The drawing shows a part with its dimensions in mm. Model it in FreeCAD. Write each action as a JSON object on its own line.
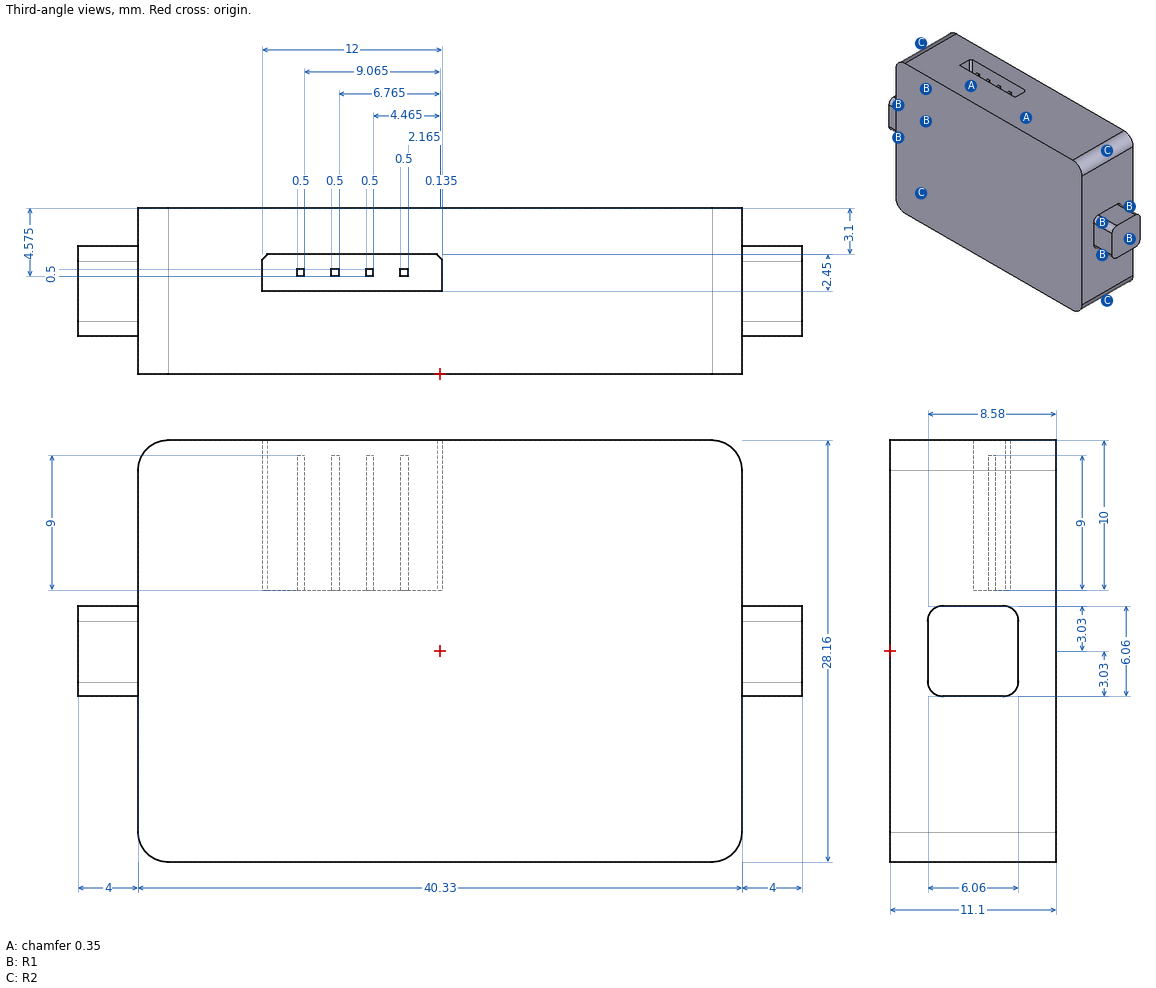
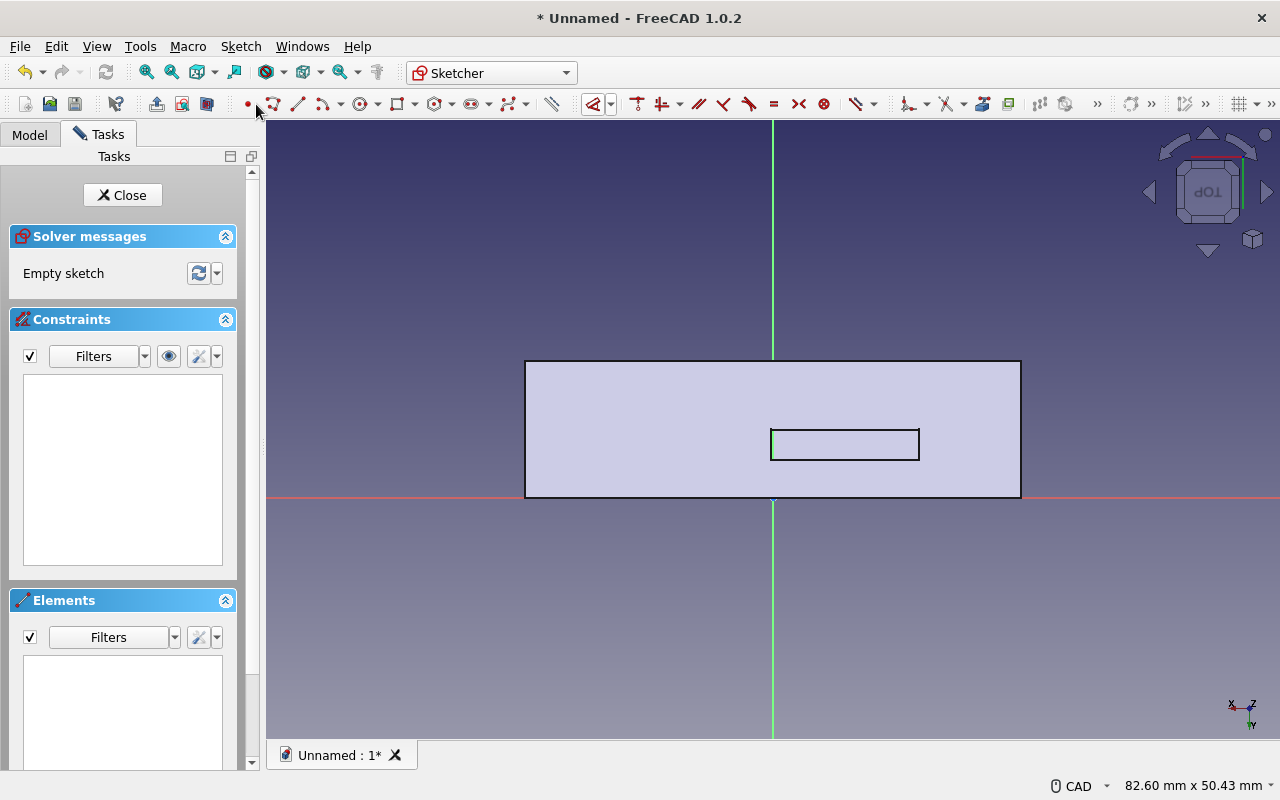
{"action": "scroll", "coordinate": [838, 445], "scroll_direction": "up", "scroll_amount": 15}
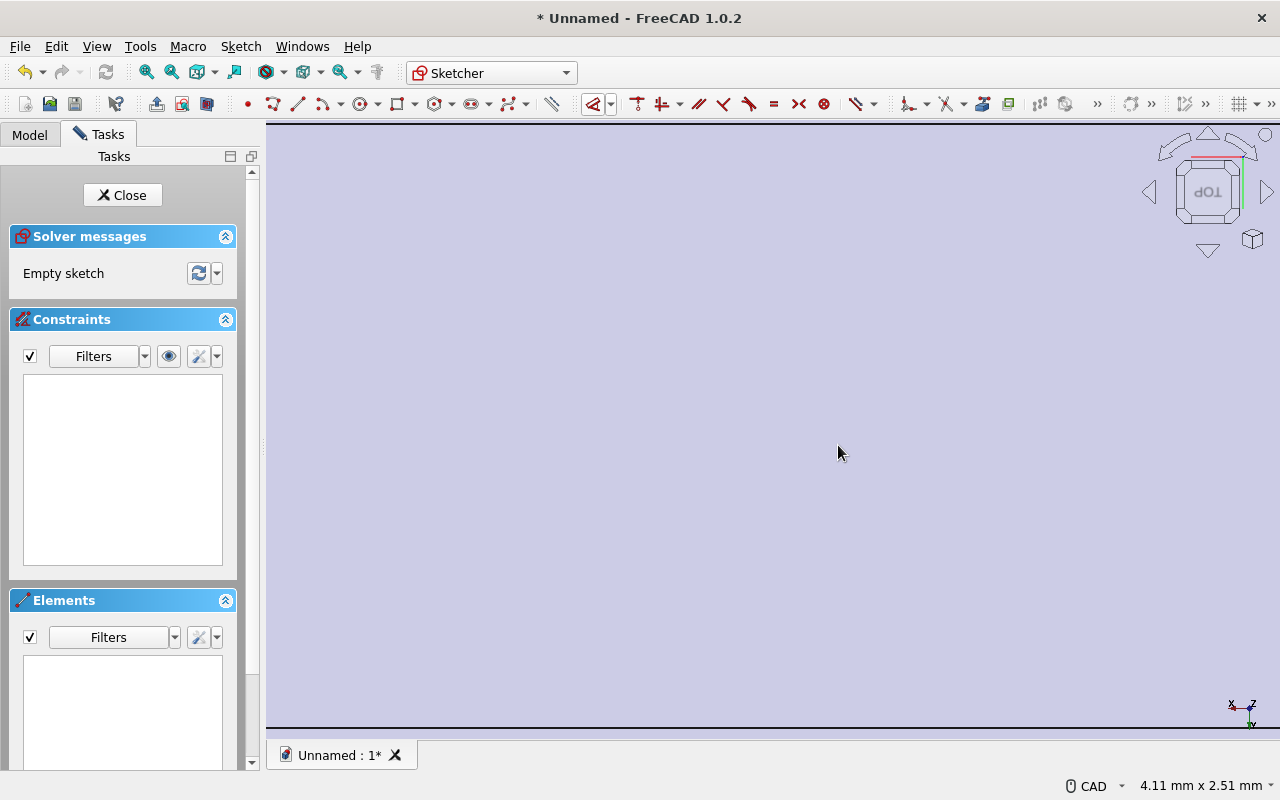
{"action": "scroll", "coordinate": [675, 424], "scroll_direction": "up", "scroll_amount": 6}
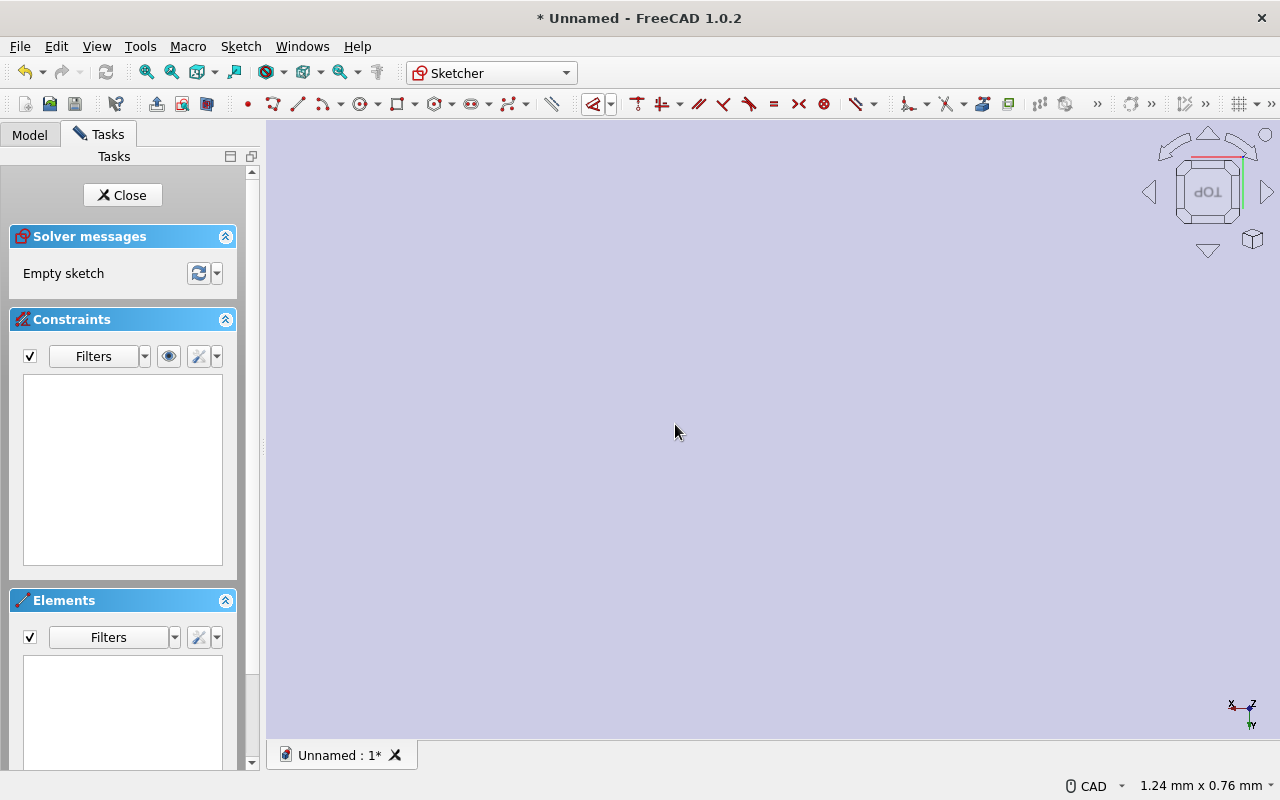
{"action": "key", "text": "g r"}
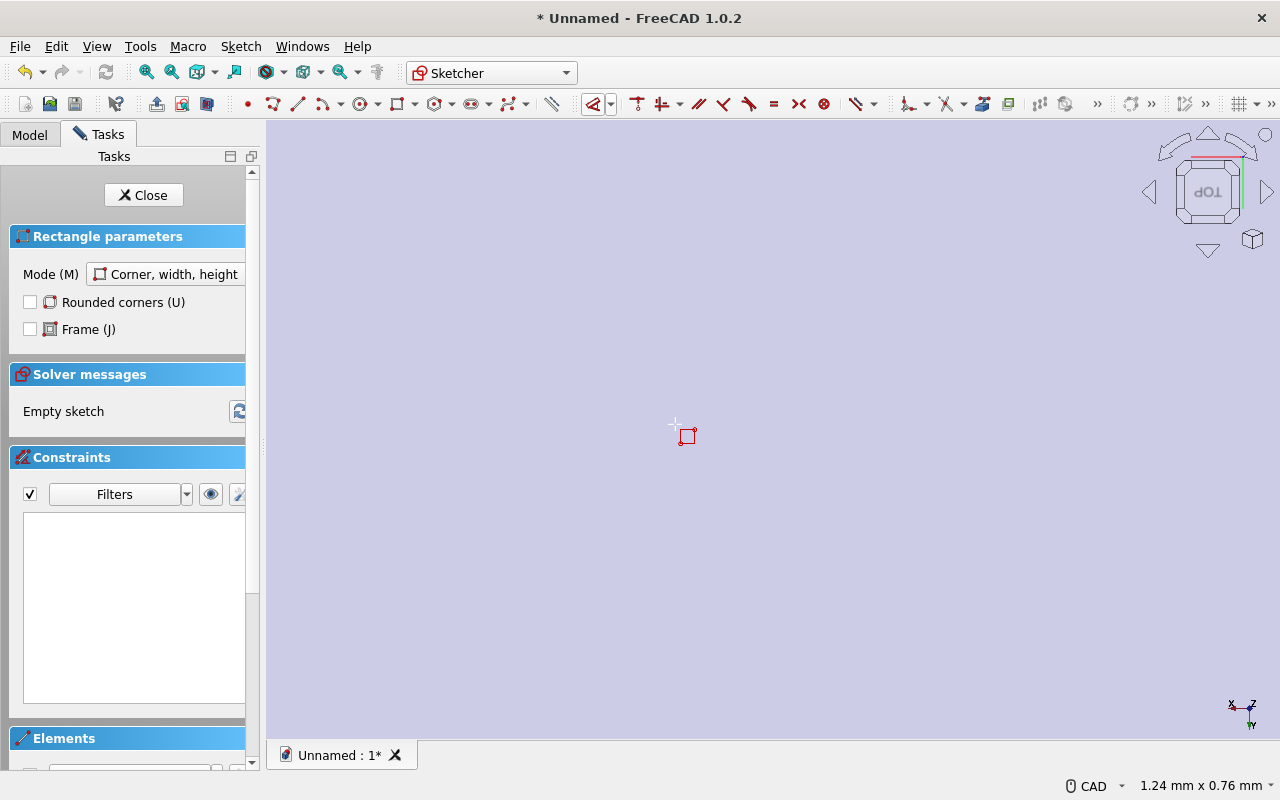
{"action": "left_click", "coordinate": [500, 224]}
{"action": "mouse_move", "coordinate": [909, 633]}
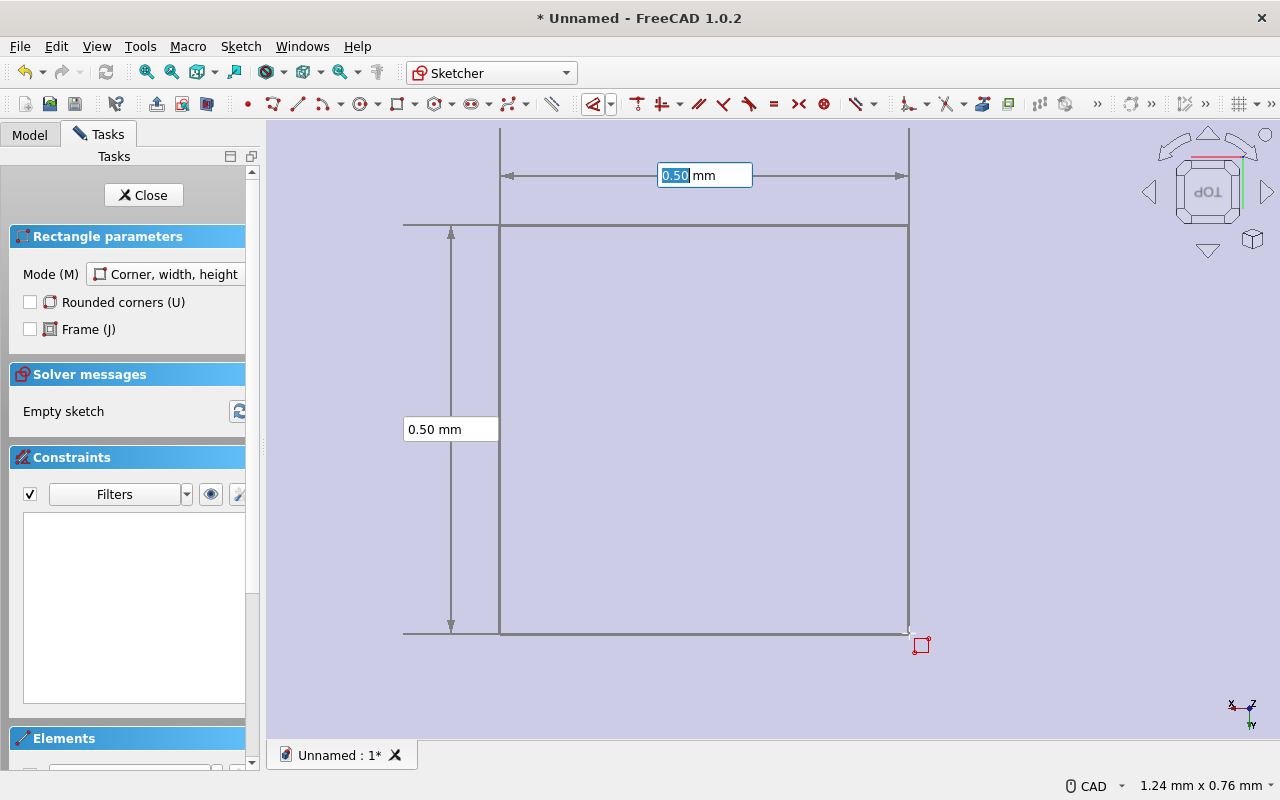
{"action": "type", "text": "0.5"}
{"action": "key", "text": "Tab"}
{"action": "type", "text": "0.5"}
{"action": "key", "text": "Return"}
{"action": "key", "text": "Escape"}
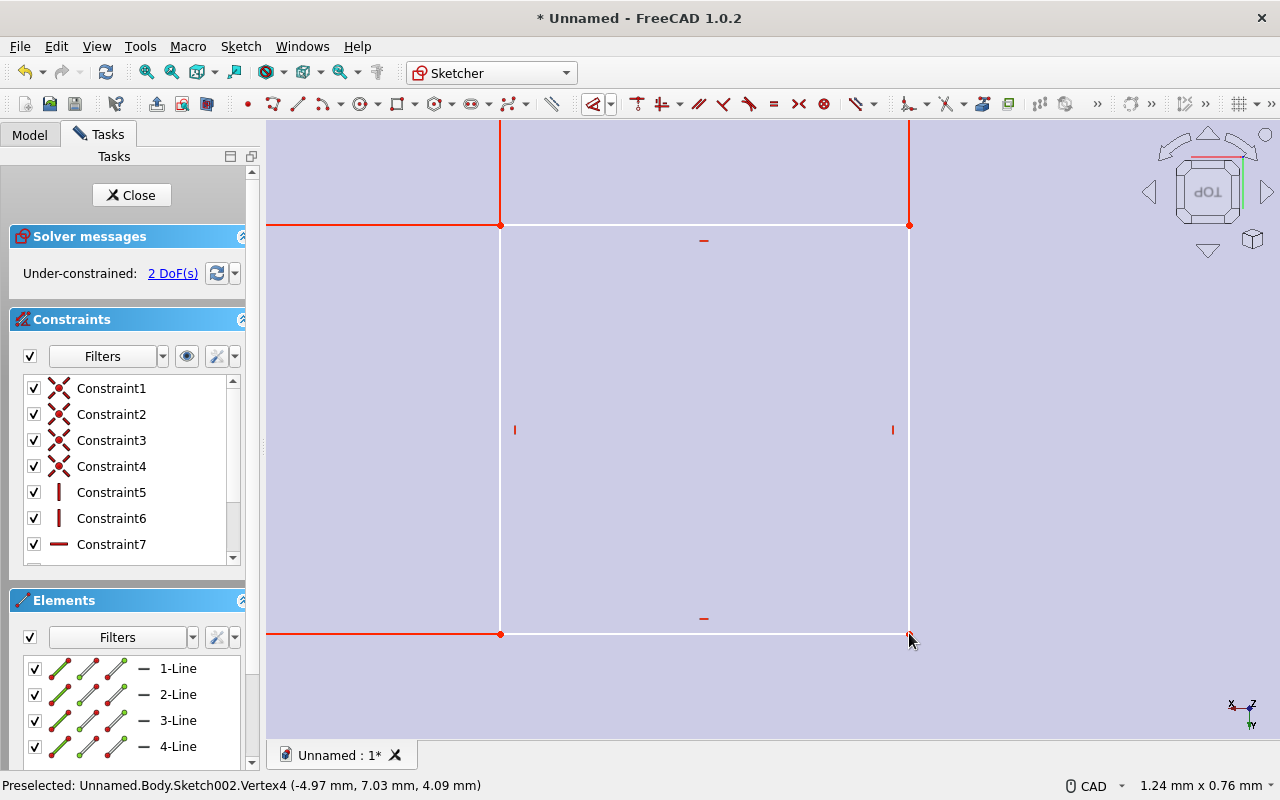
{"action": "left_click", "coordinate": [592, 104]}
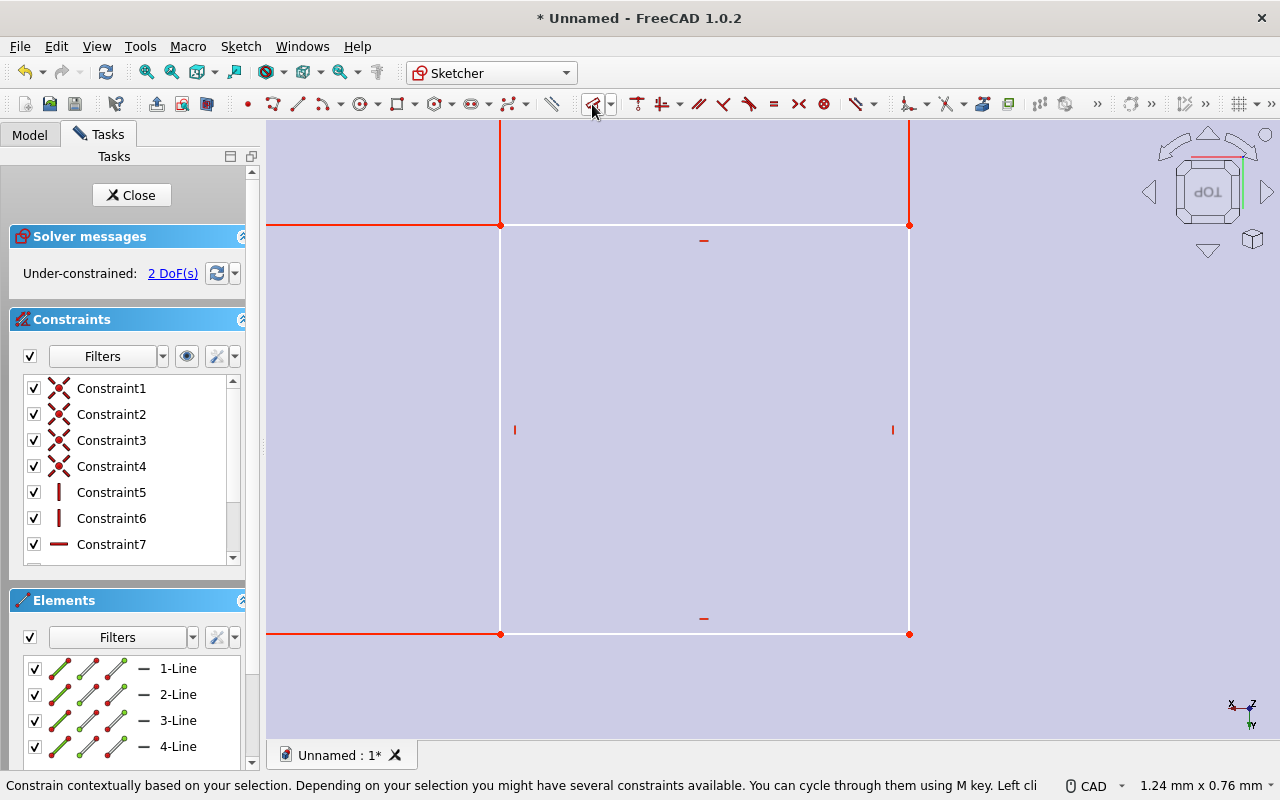
{"action": "left_click", "coordinate": [500, 225]}
{"action": "left_click", "coordinate": [397, 191]}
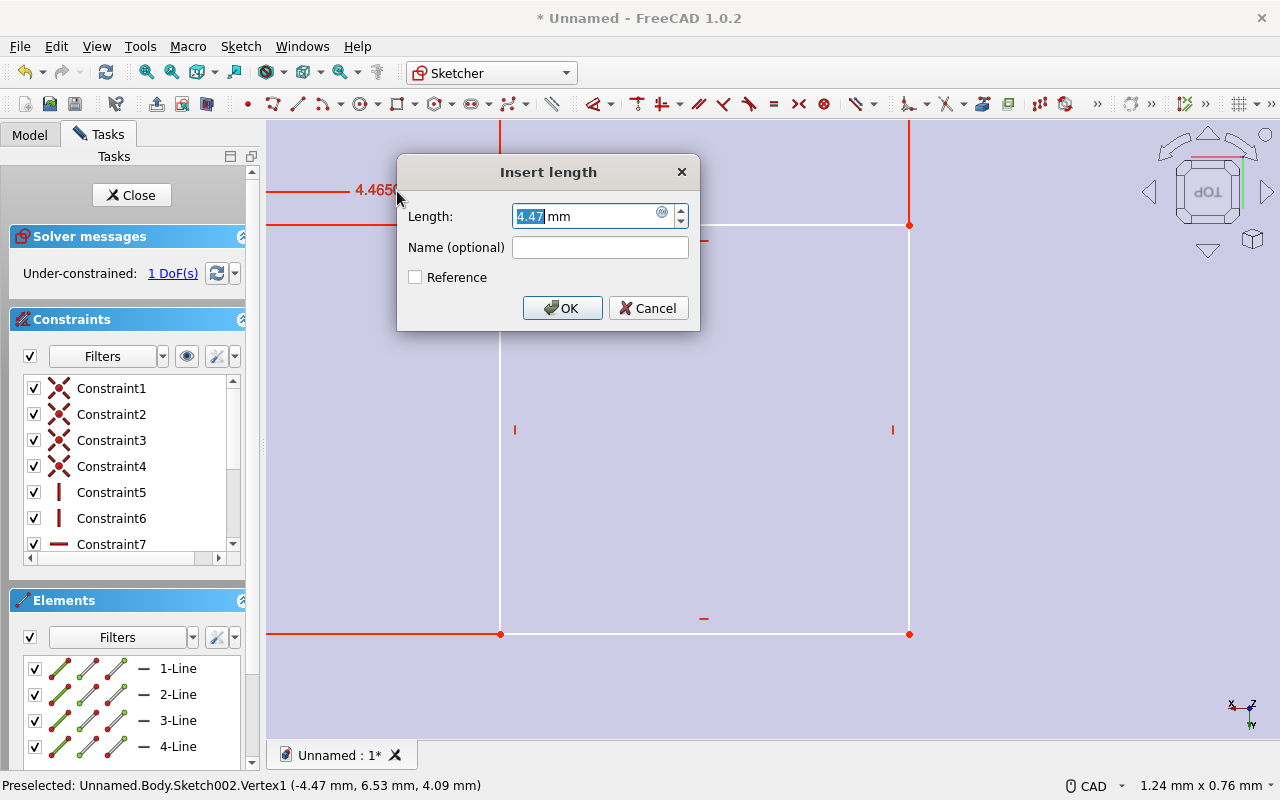
{"action": "type", "text": "4.465"}
{"action": "key", "text": "Return"}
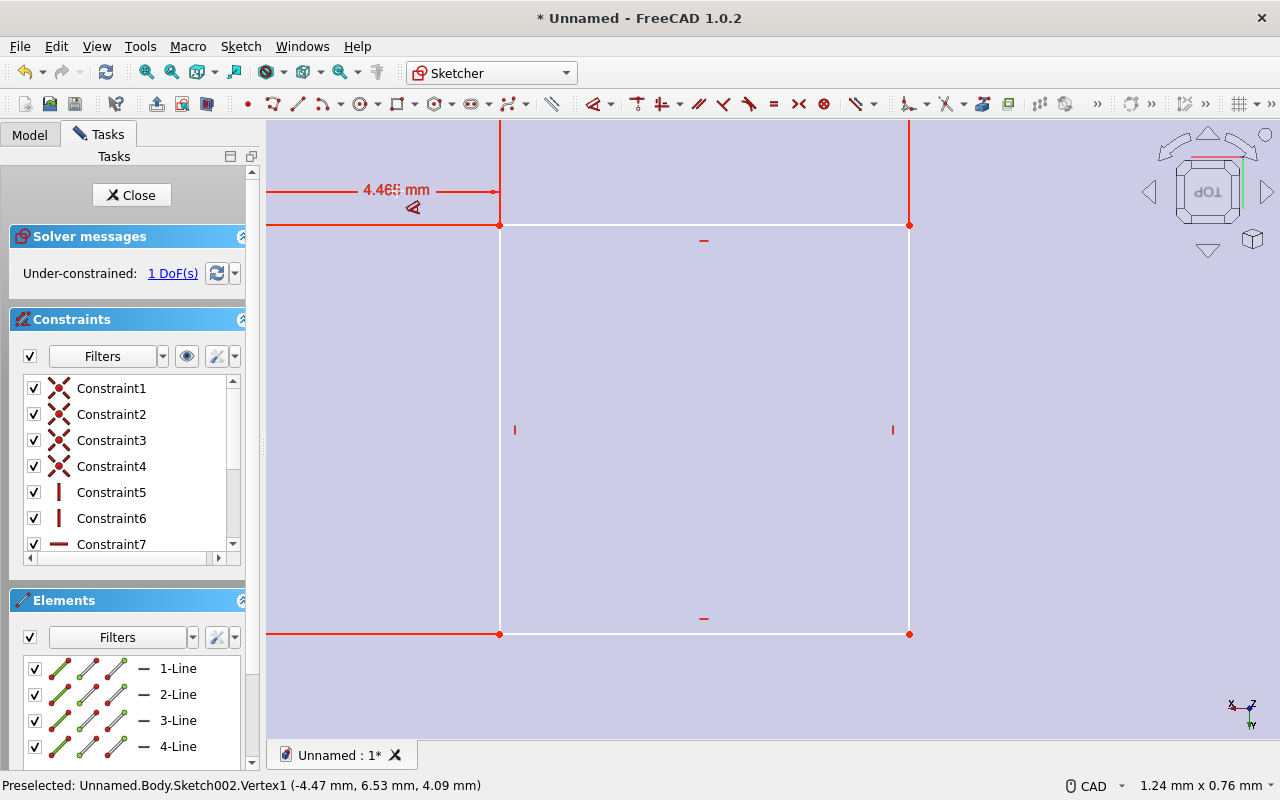
{"action": "left_click", "coordinate": [500, 225]}
{"action": "left_click", "coordinate": [534, 468]}